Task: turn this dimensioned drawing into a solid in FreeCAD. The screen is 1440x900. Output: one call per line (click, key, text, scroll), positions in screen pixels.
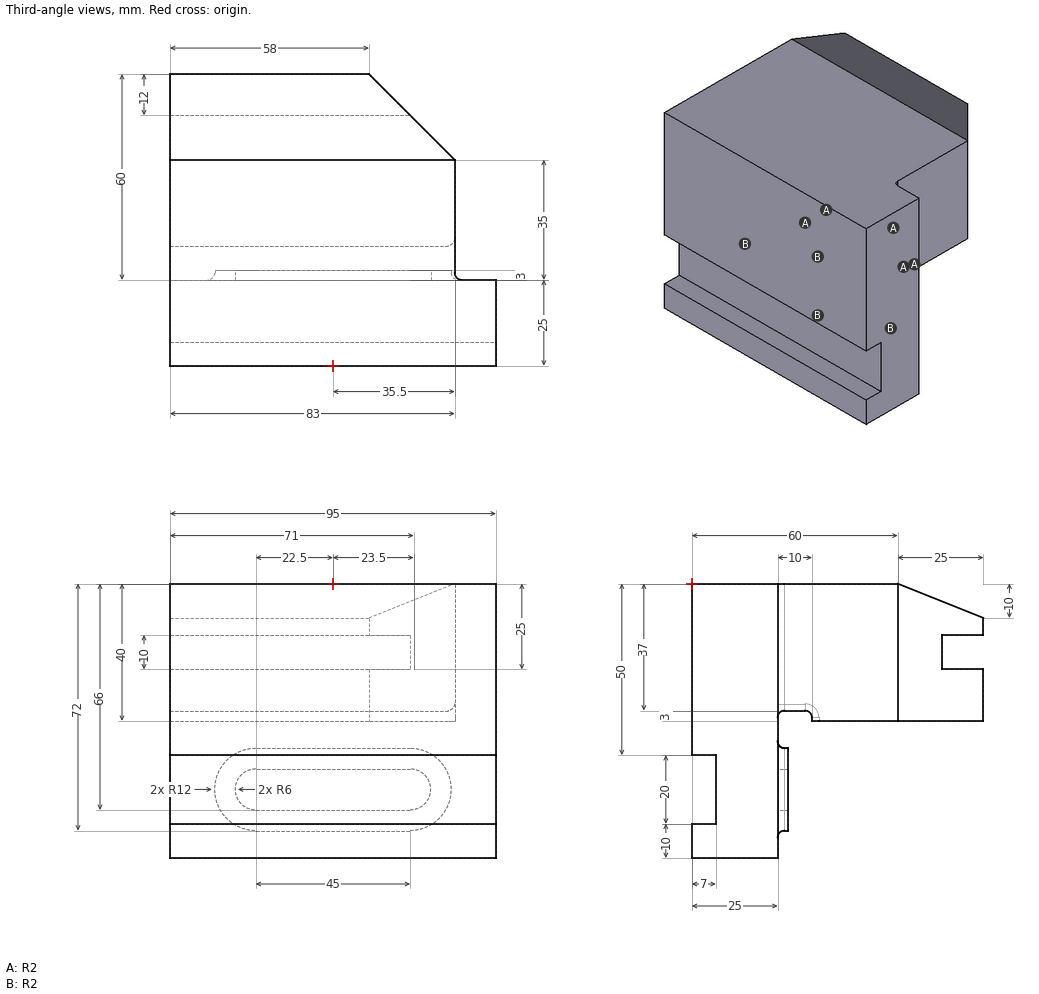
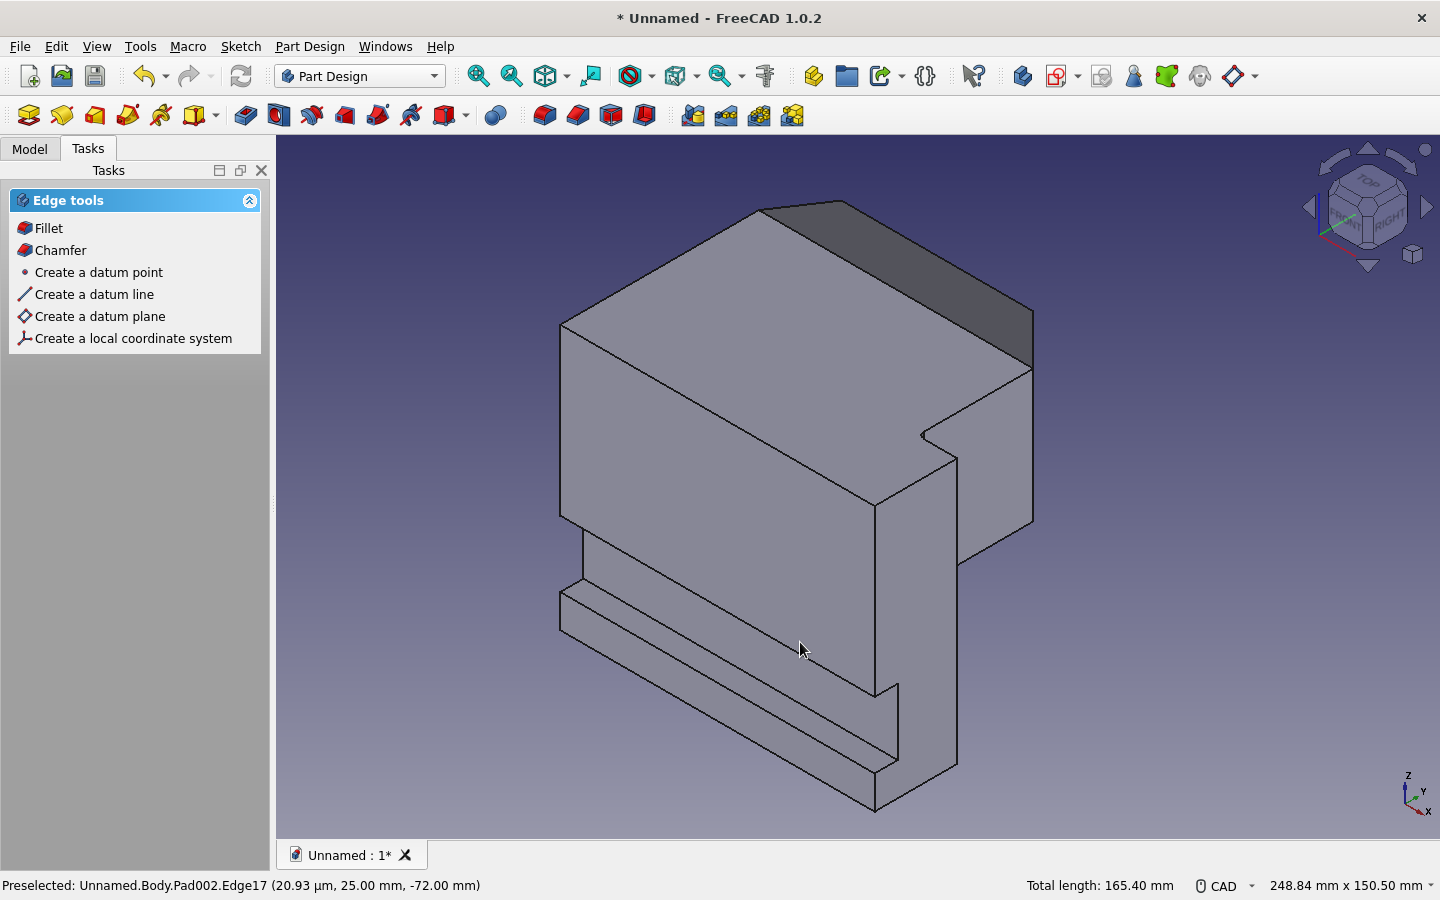
click(545, 116)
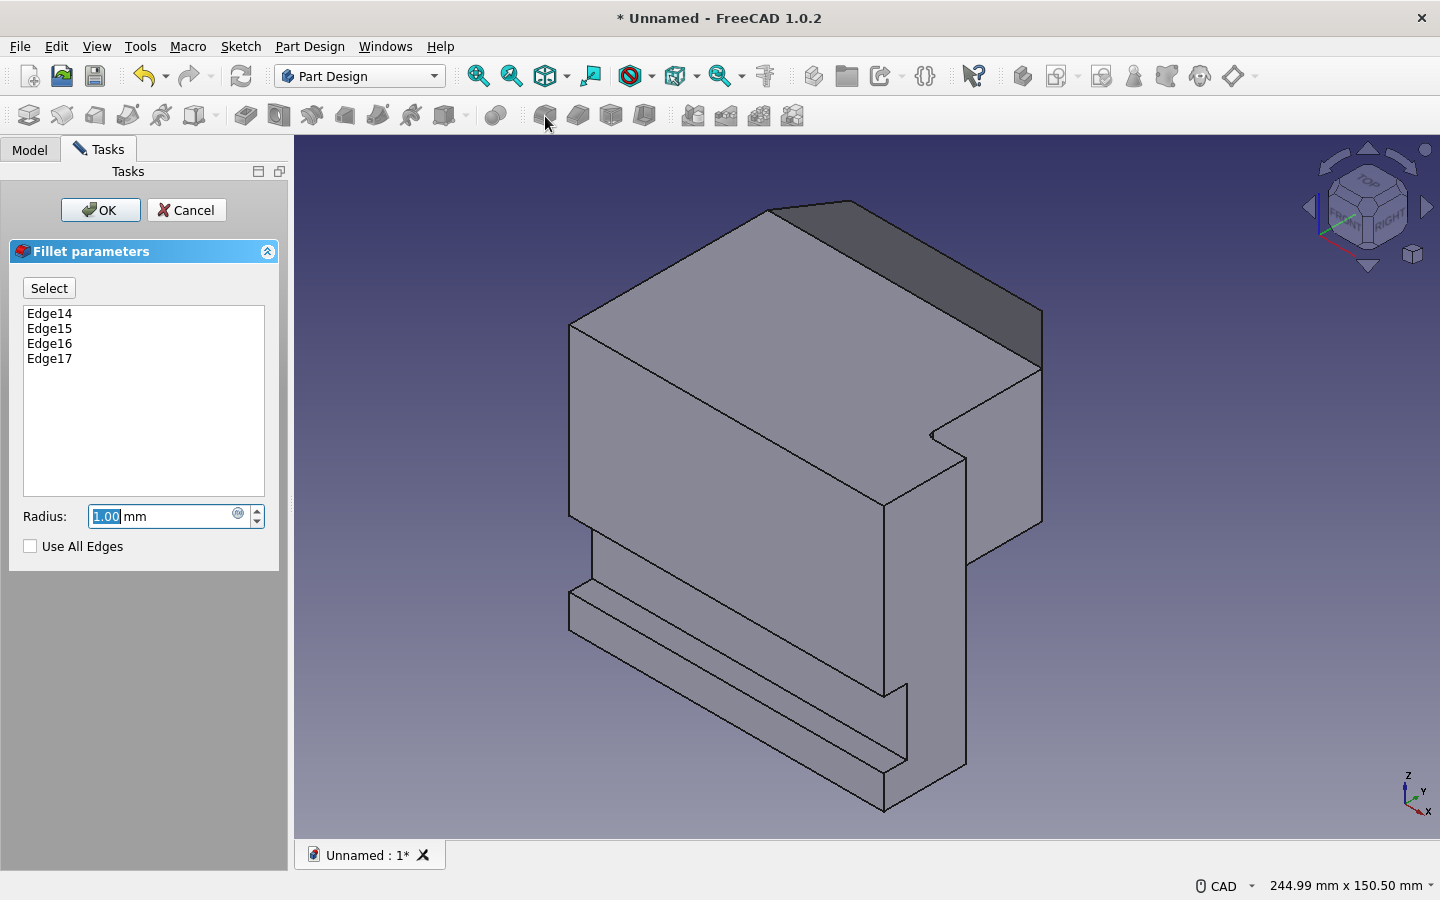
text(2)
key(Tab)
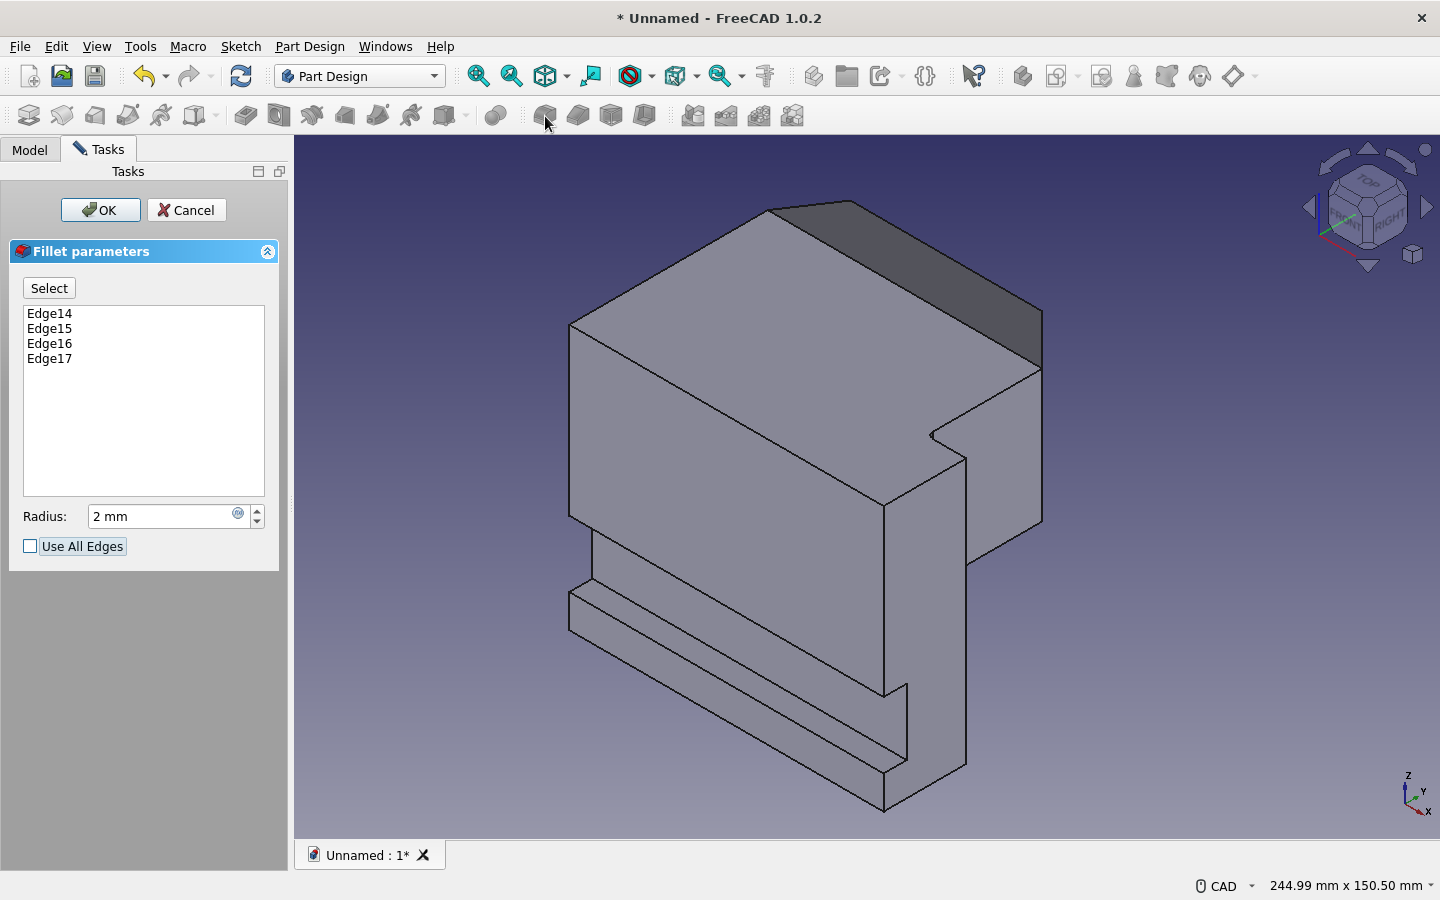
click(101, 210)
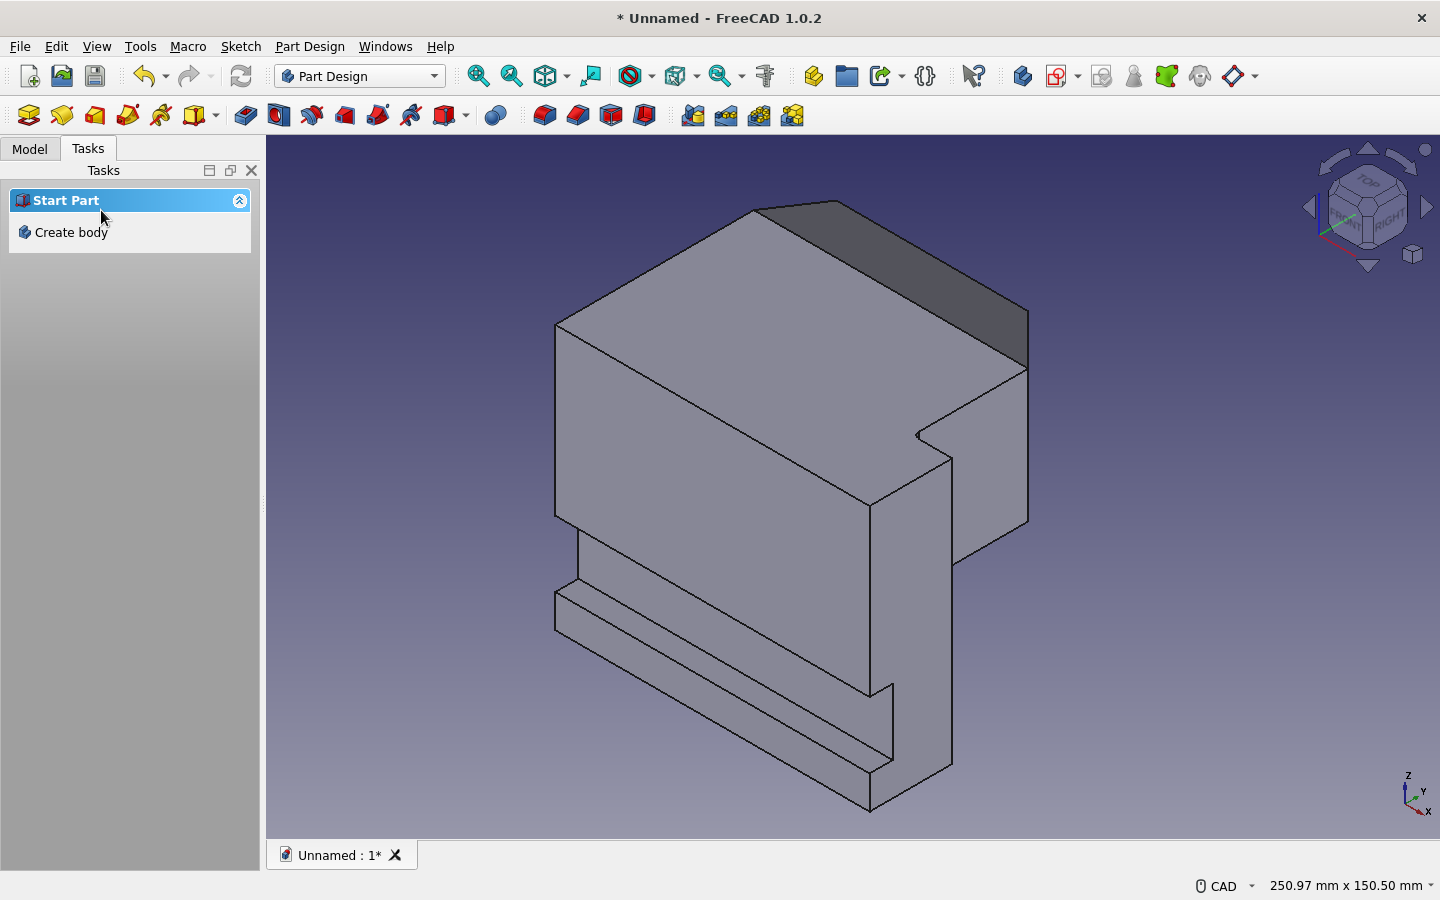
key(4)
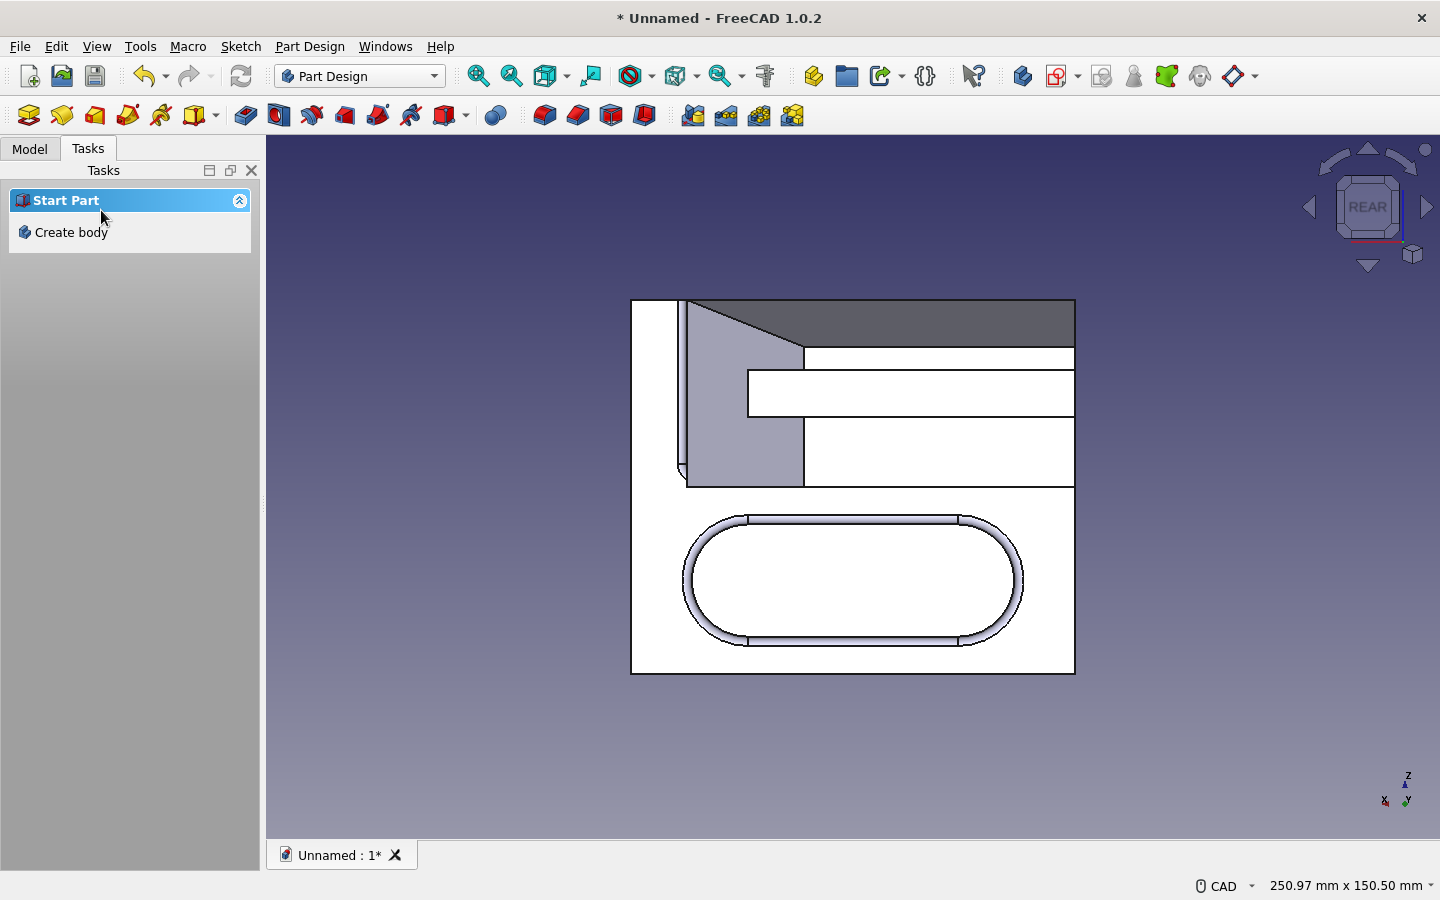
click(761, 580)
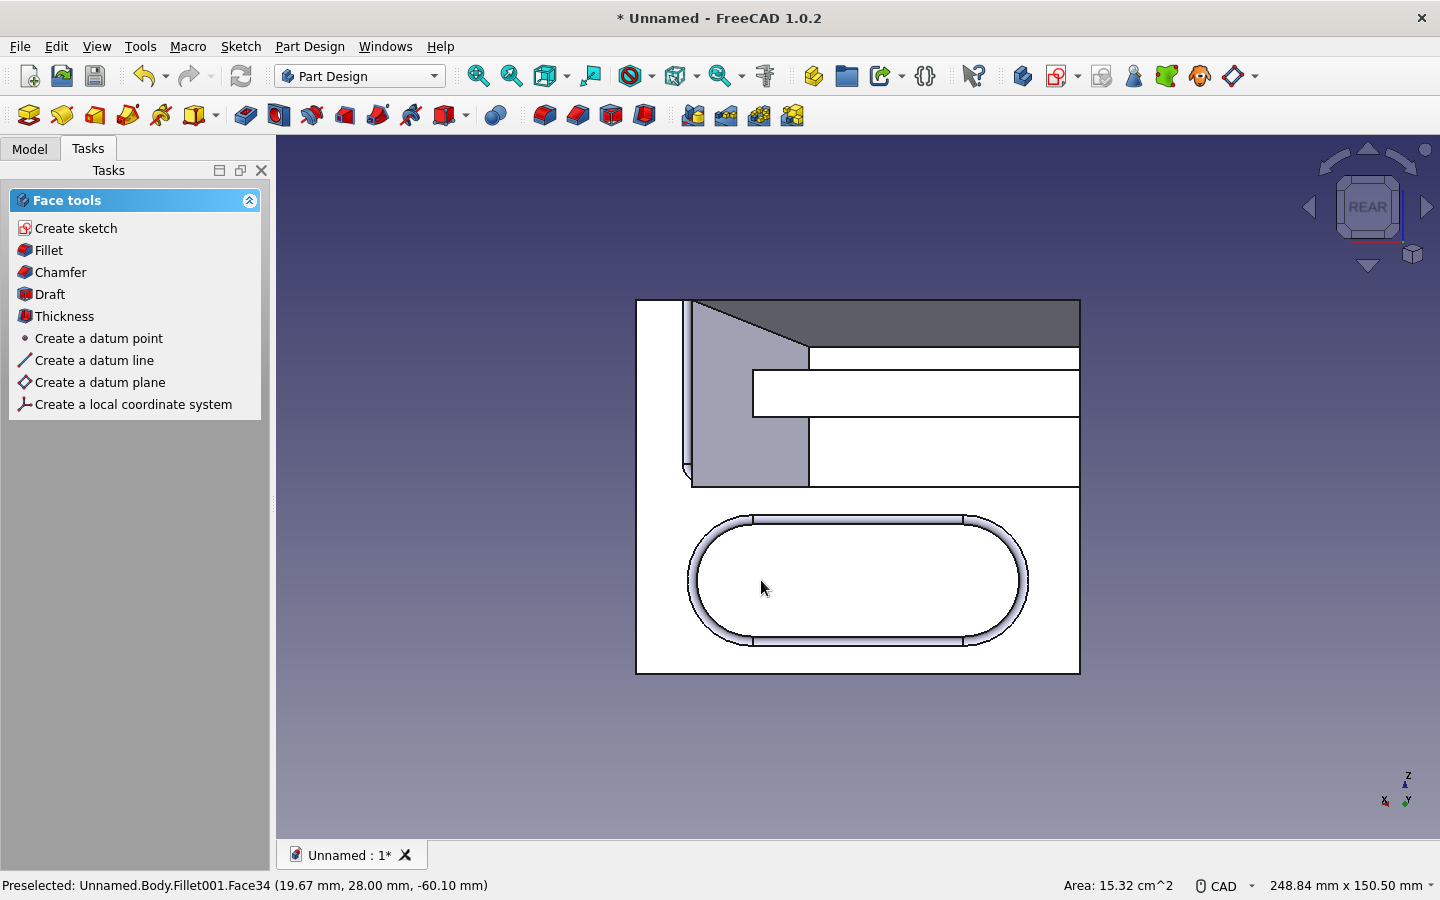
click(1056, 76)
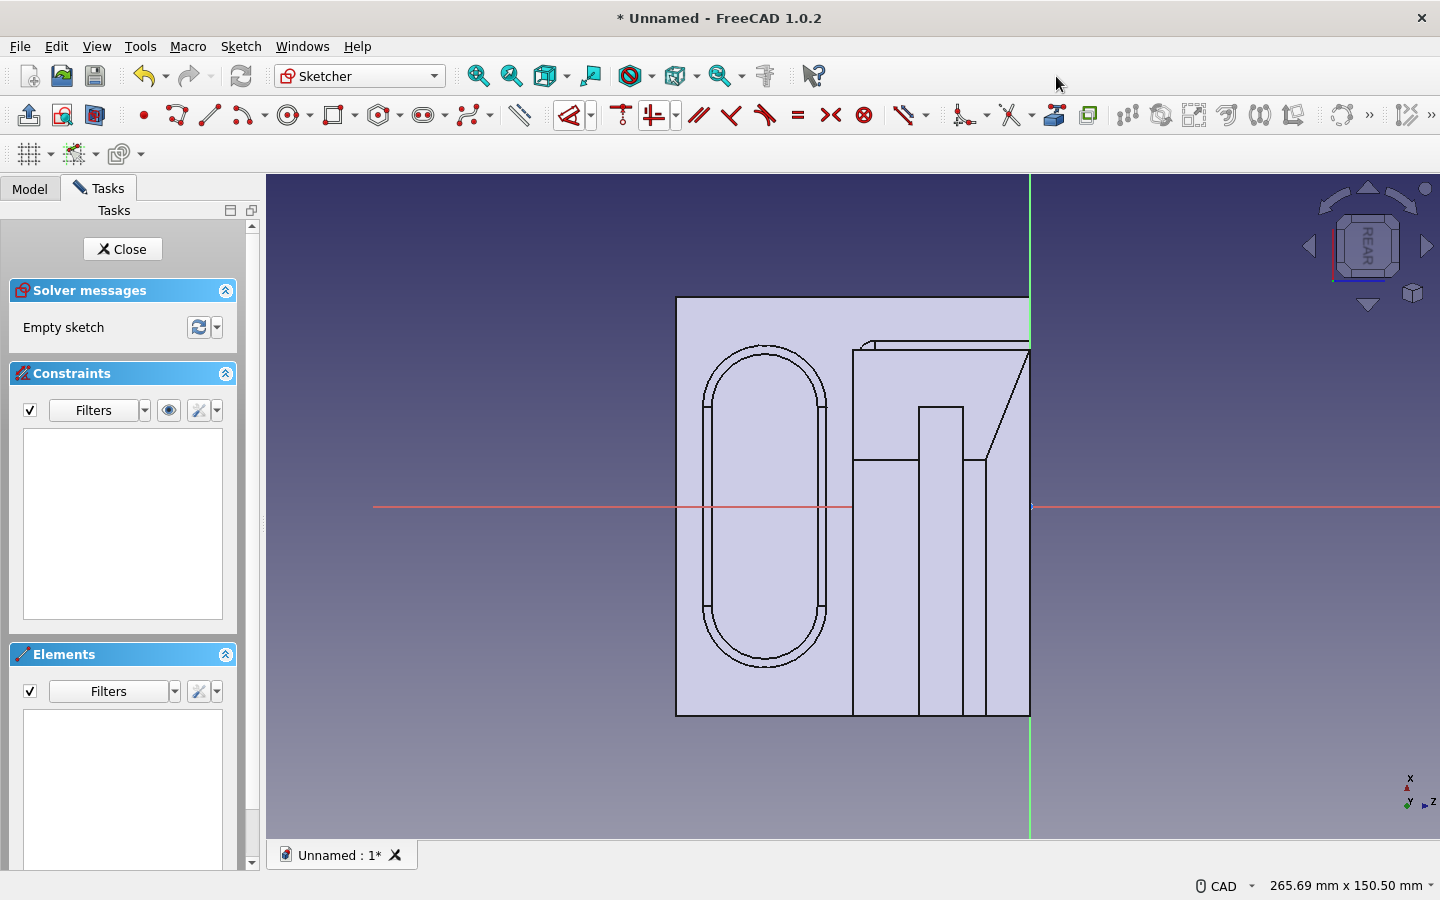
click(95, 116)